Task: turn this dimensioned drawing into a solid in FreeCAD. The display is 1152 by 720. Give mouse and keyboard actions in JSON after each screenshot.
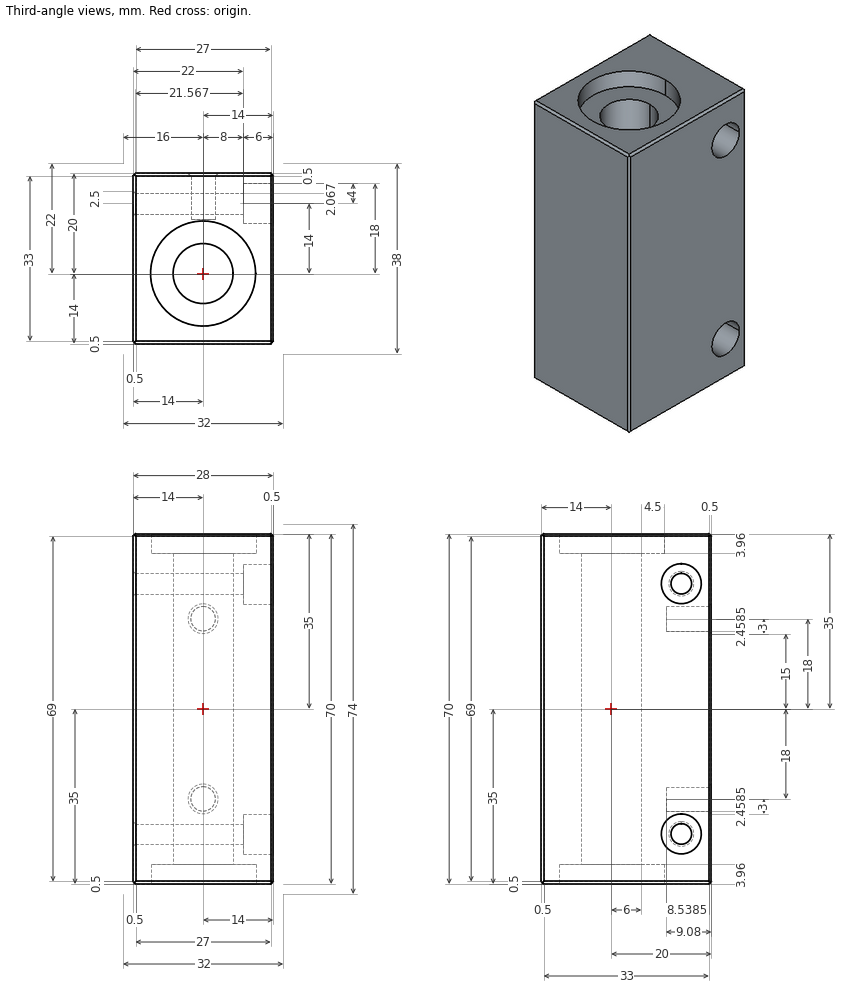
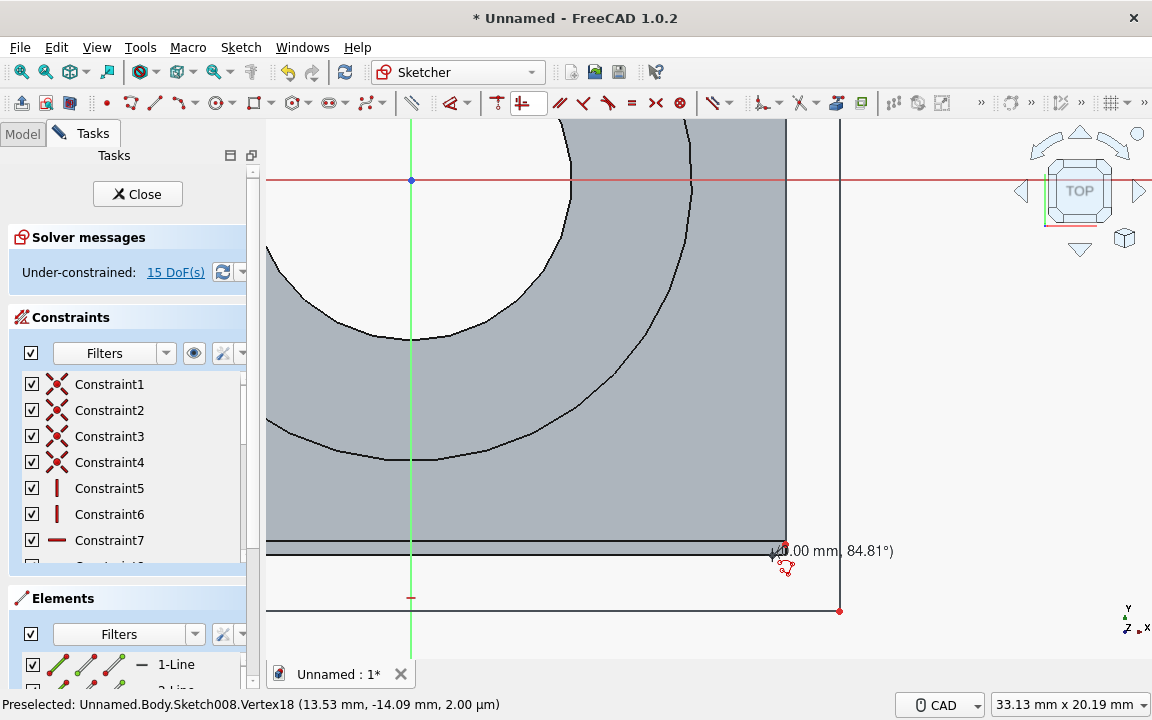
{"action": "scroll", "coordinate": [774, 557], "scroll_direction": "down", "scroll_amount": 5}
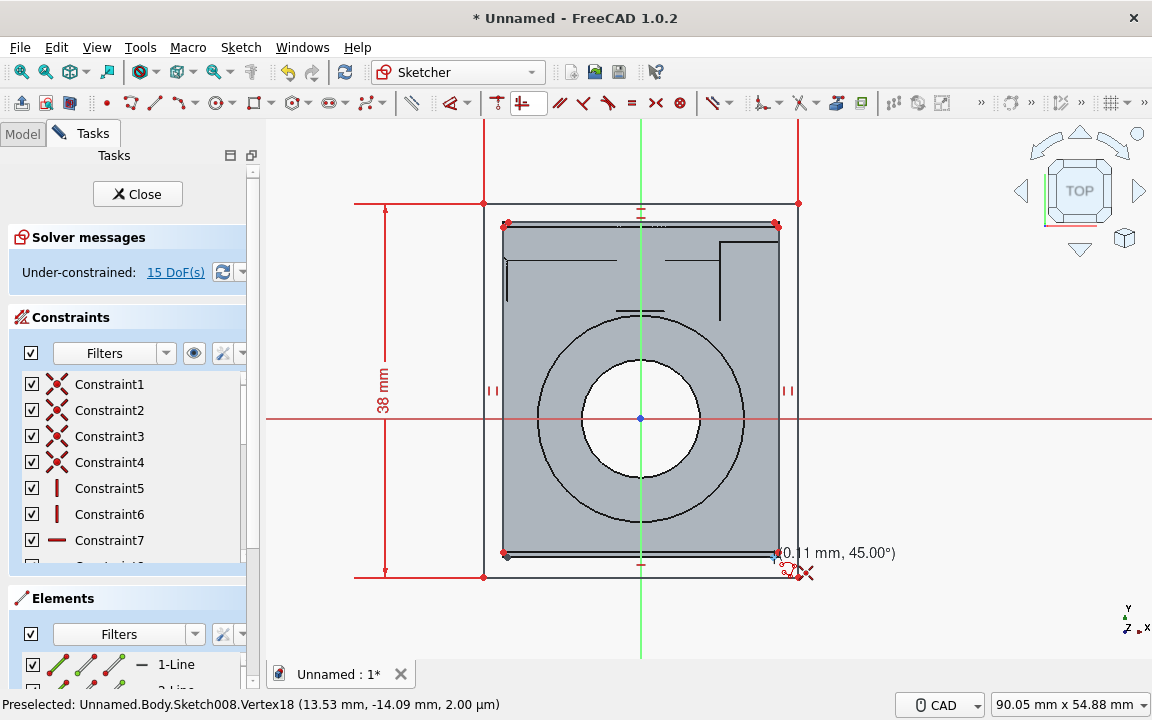
{"action": "scroll", "coordinate": [508, 557], "scroll_direction": "up", "scroll_amount": 8}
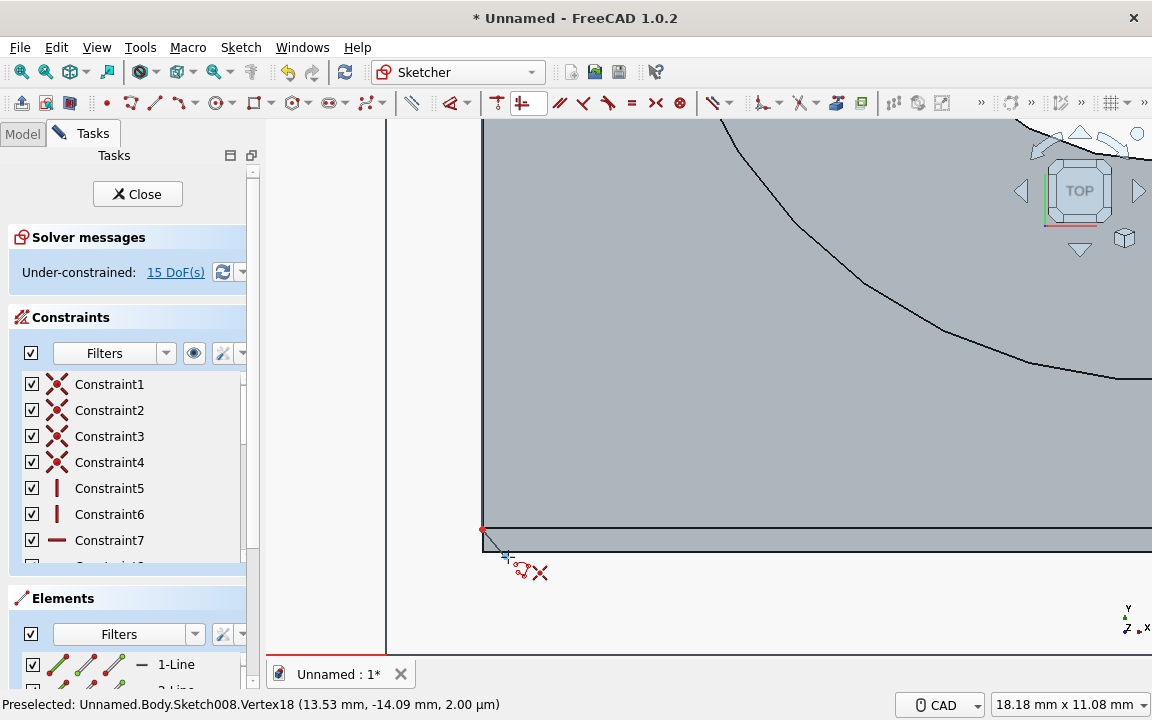
{"action": "left_click", "coordinate": [505, 557]}
{"action": "key", "text": "Escape"}
{"action": "key", "text": "Escape"}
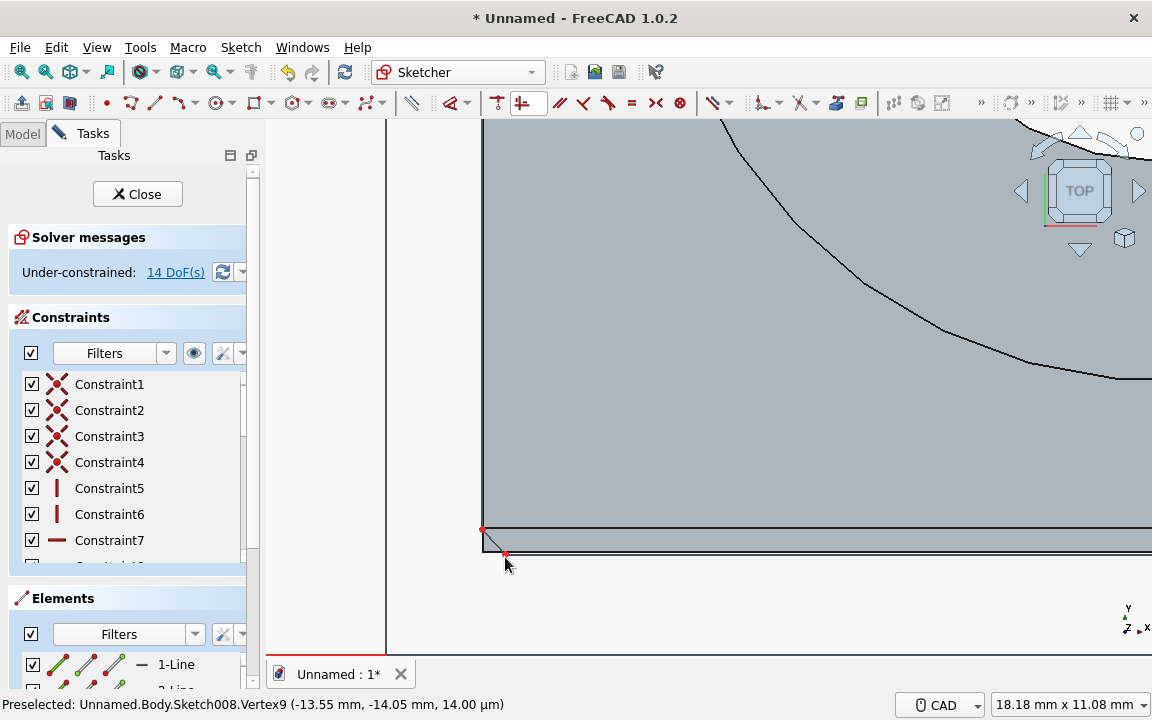
{"action": "left_click", "coordinate": [450, 104]}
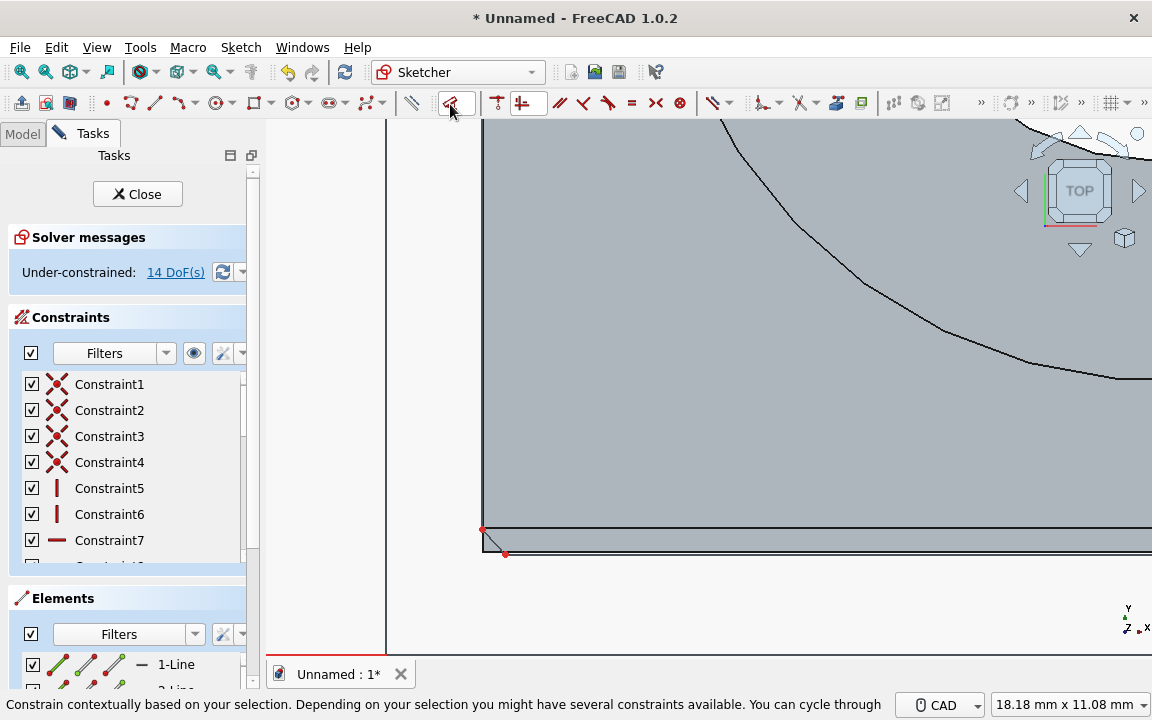
{"action": "scroll", "coordinate": [508, 557], "scroll_direction": "down", "scroll_amount": 8}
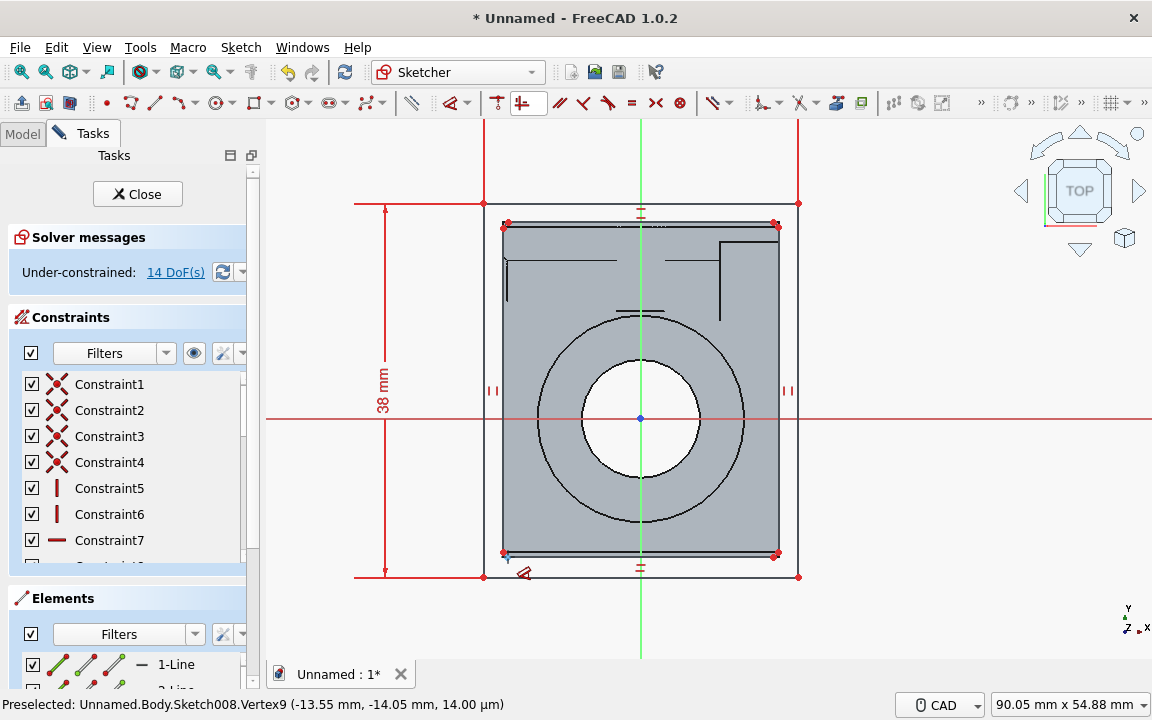
{"action": "left_click", "coordinate": [503, 487]}
{"action": "left_click", "coordinate": [469, 390]}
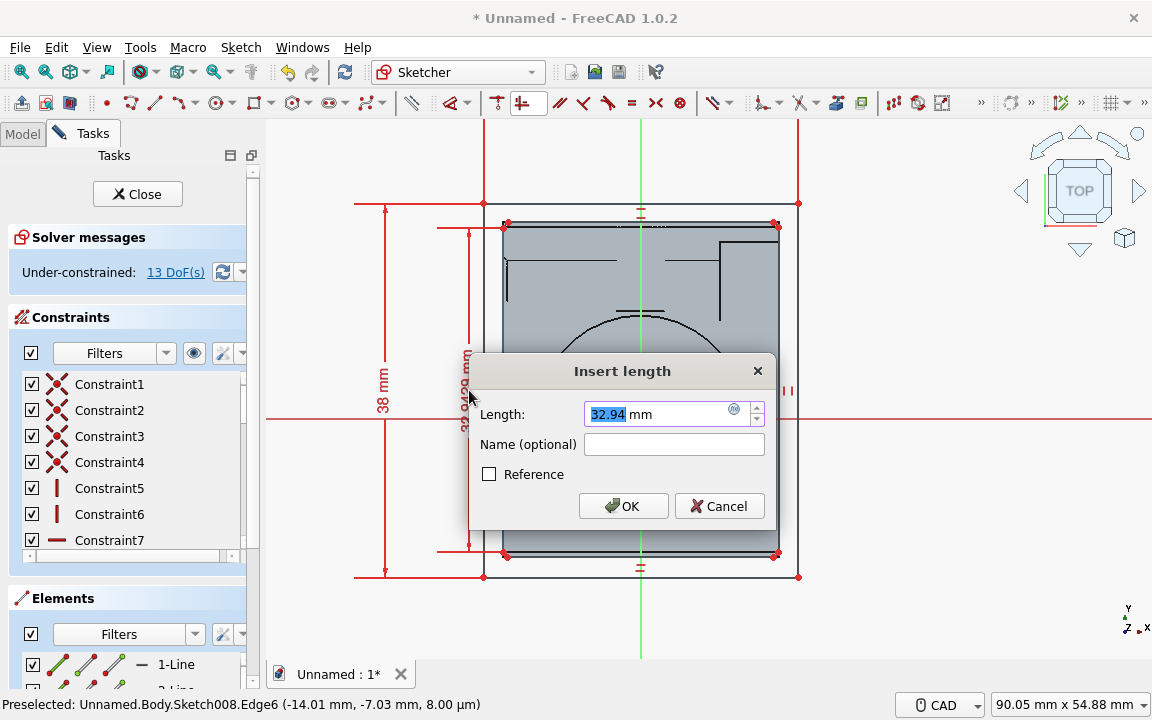
{"action": "type", "text": "33"}
{"action": "key", "text": "Return"}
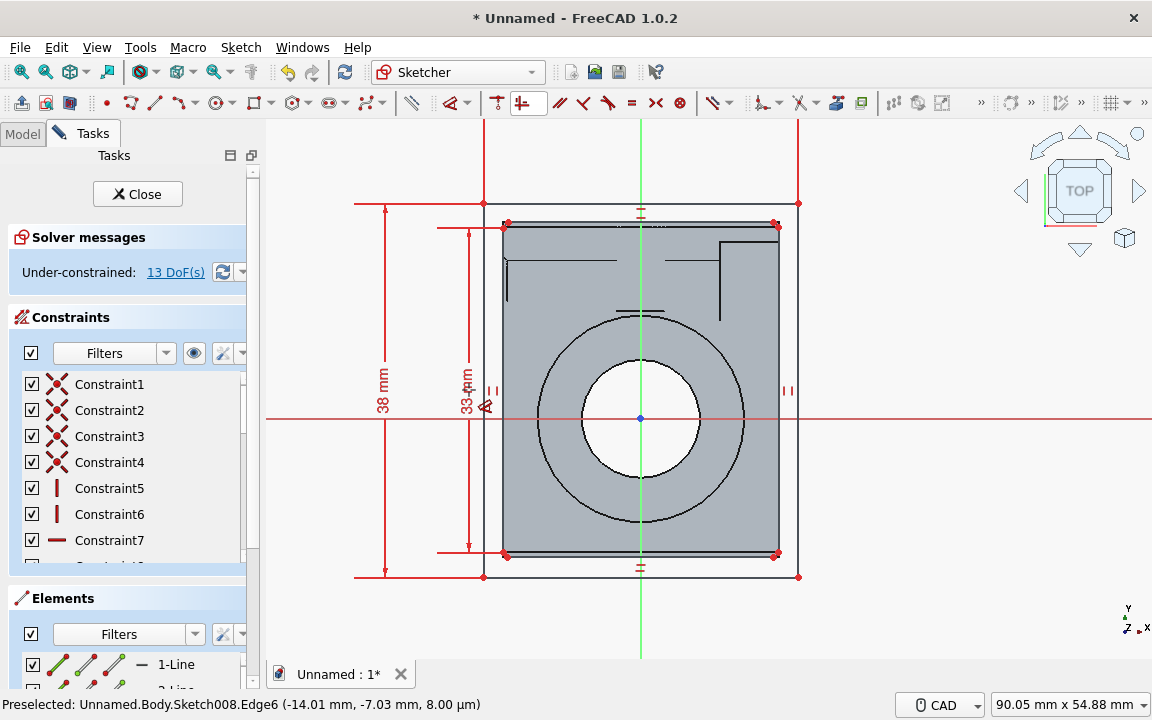
{"action": "left_click", "coordinate": [588, 222]}
{"action": "left_click", "coordinate": [580, 188]}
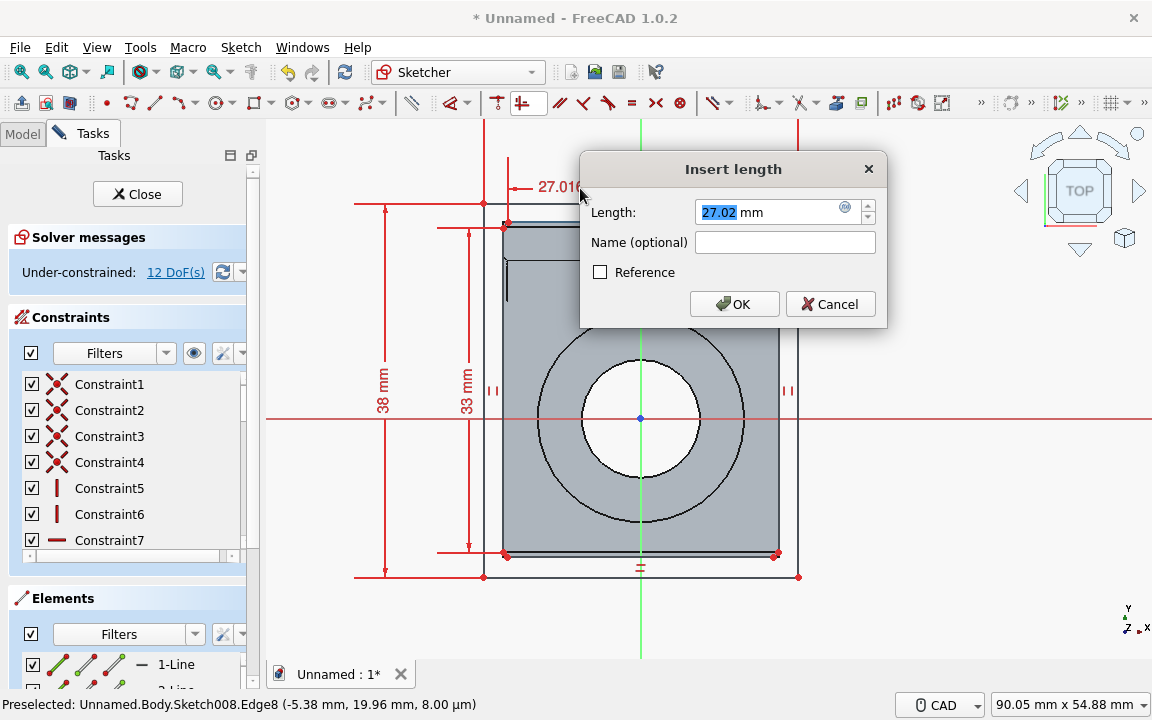
{"action": "type", "text": "27"}
{"action": "key", "text": "Return"}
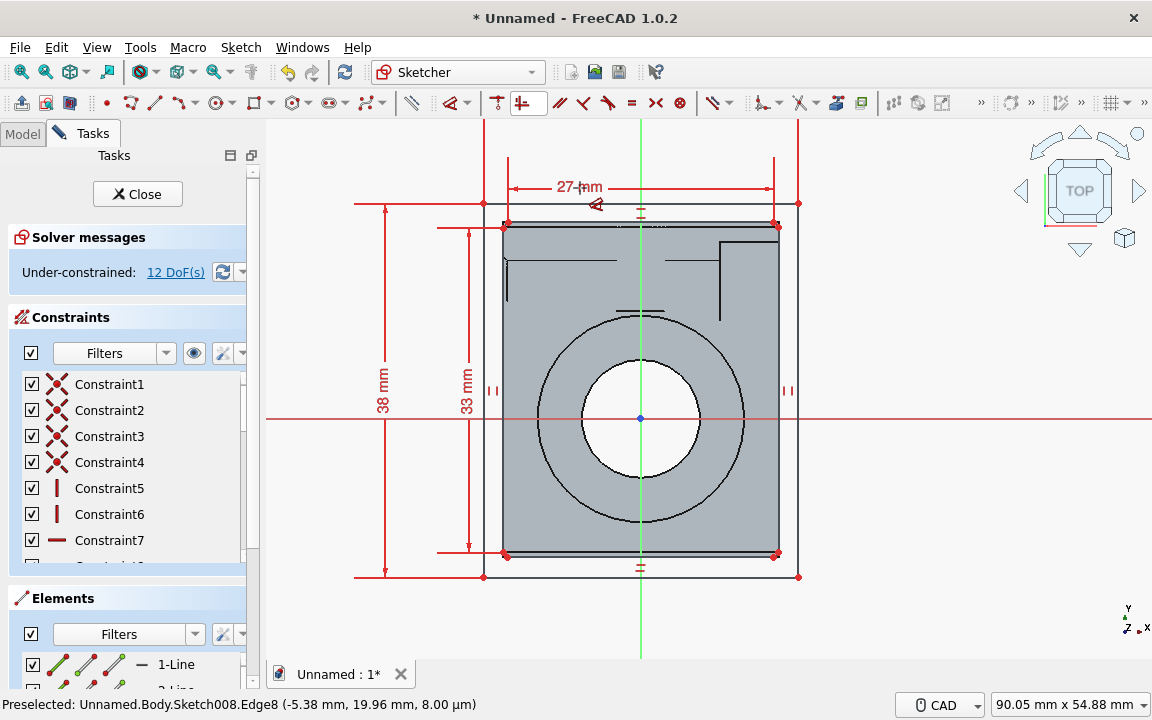
{"action": "left_click", "coordinate": [779, 325]}
{"action": "left_click", "coordinate": [813, 390]}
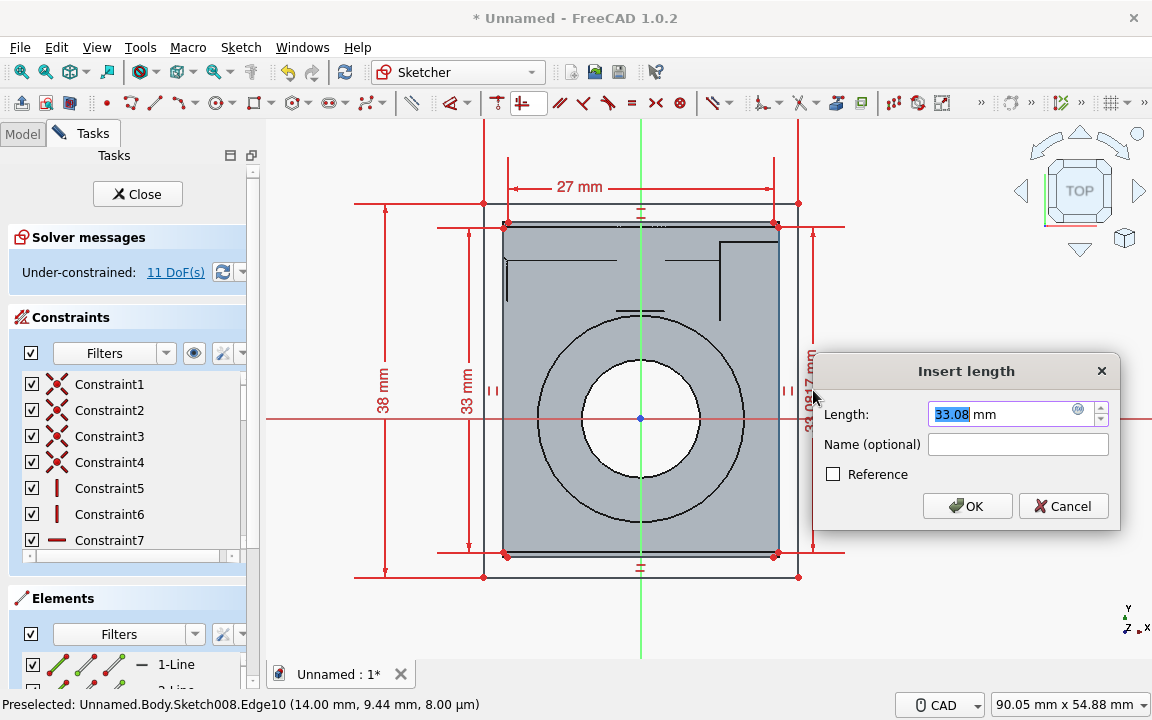
{"action": "type", "text": "33"}
{"action": "key", "text": "Return"}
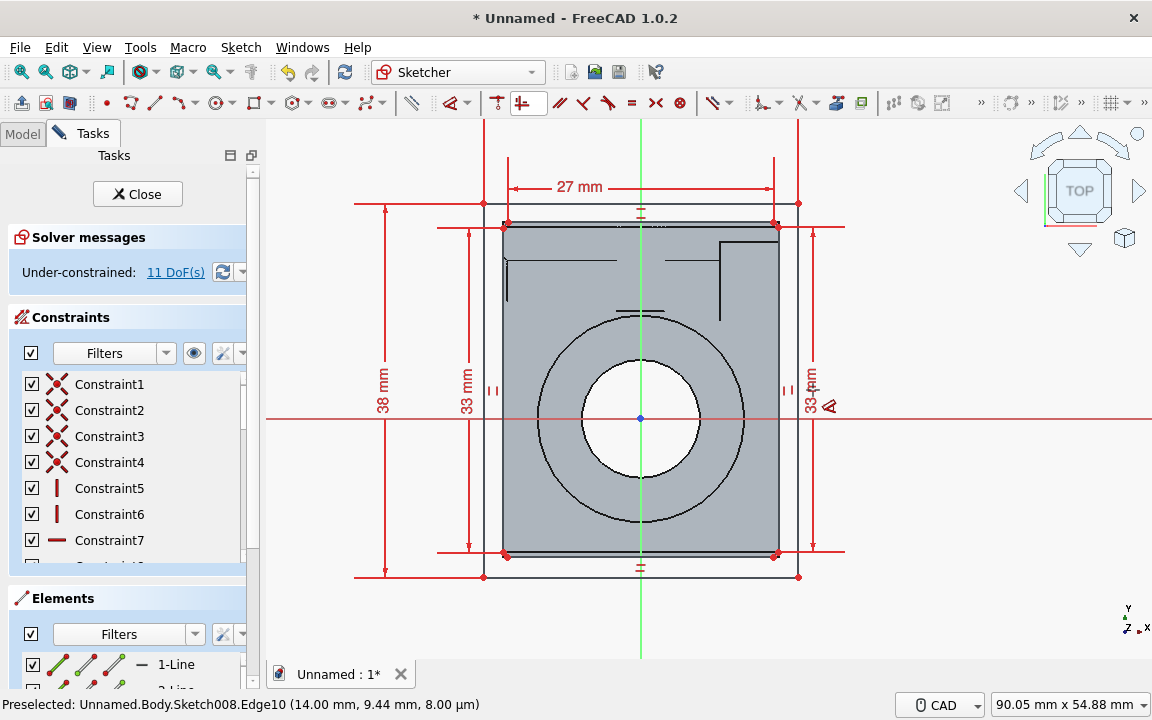
{"action": "left_click", "coordinate": [694, 557]}
{"action": "left_click", "coordinate": [579, 591]}